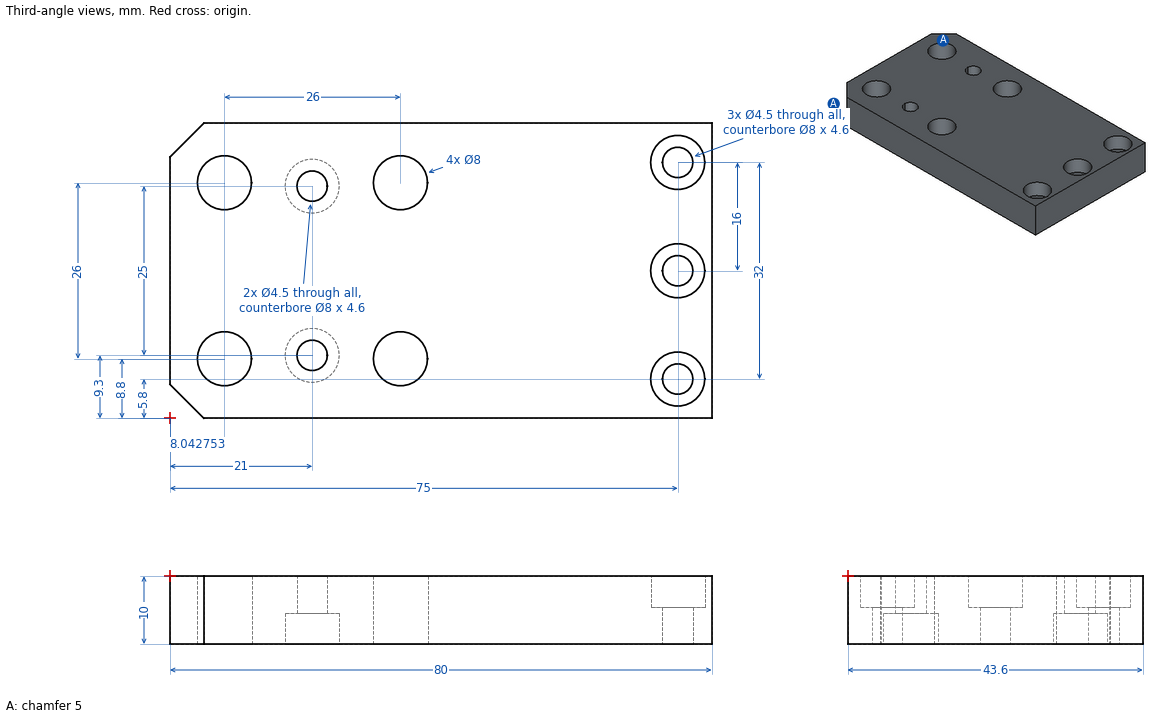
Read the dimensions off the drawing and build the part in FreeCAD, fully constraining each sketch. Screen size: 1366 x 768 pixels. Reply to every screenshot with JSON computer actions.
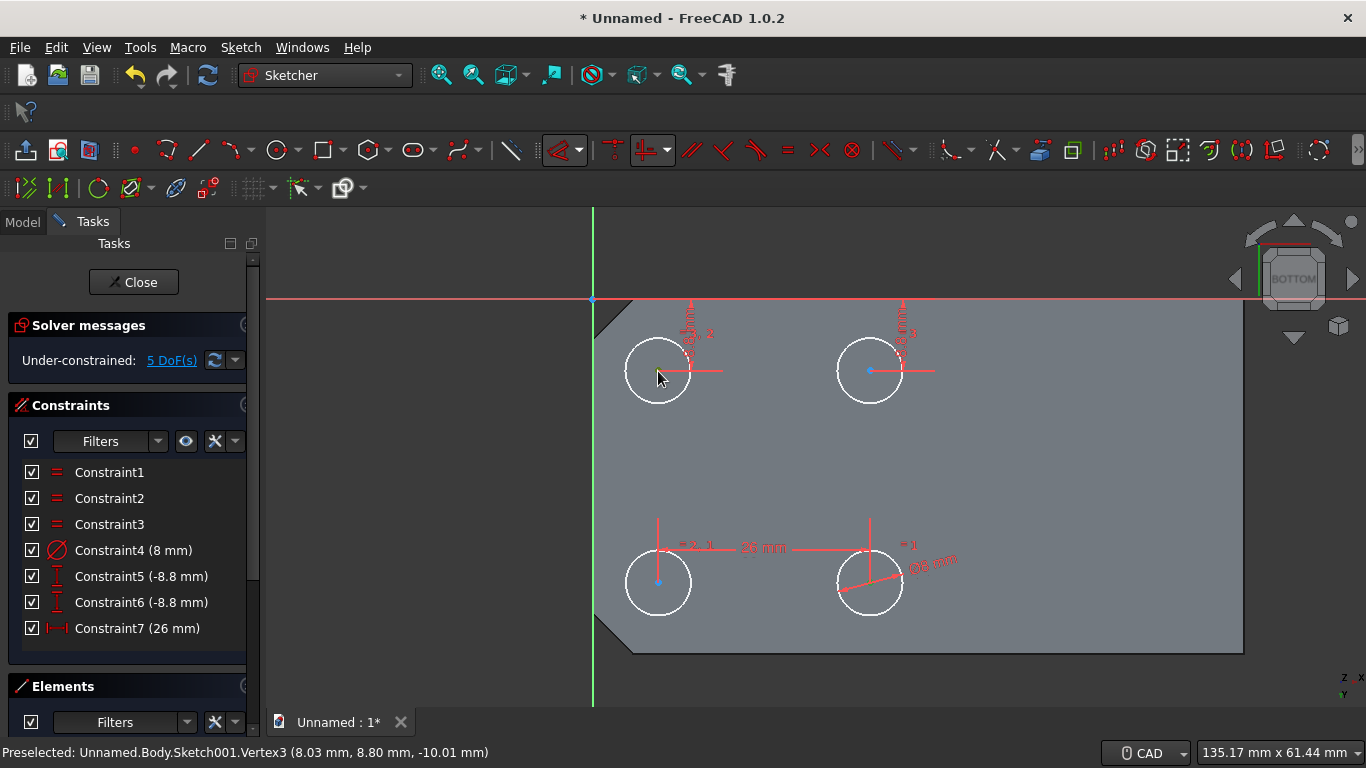
{"action": "left_click", "coordinate": [582, 150]}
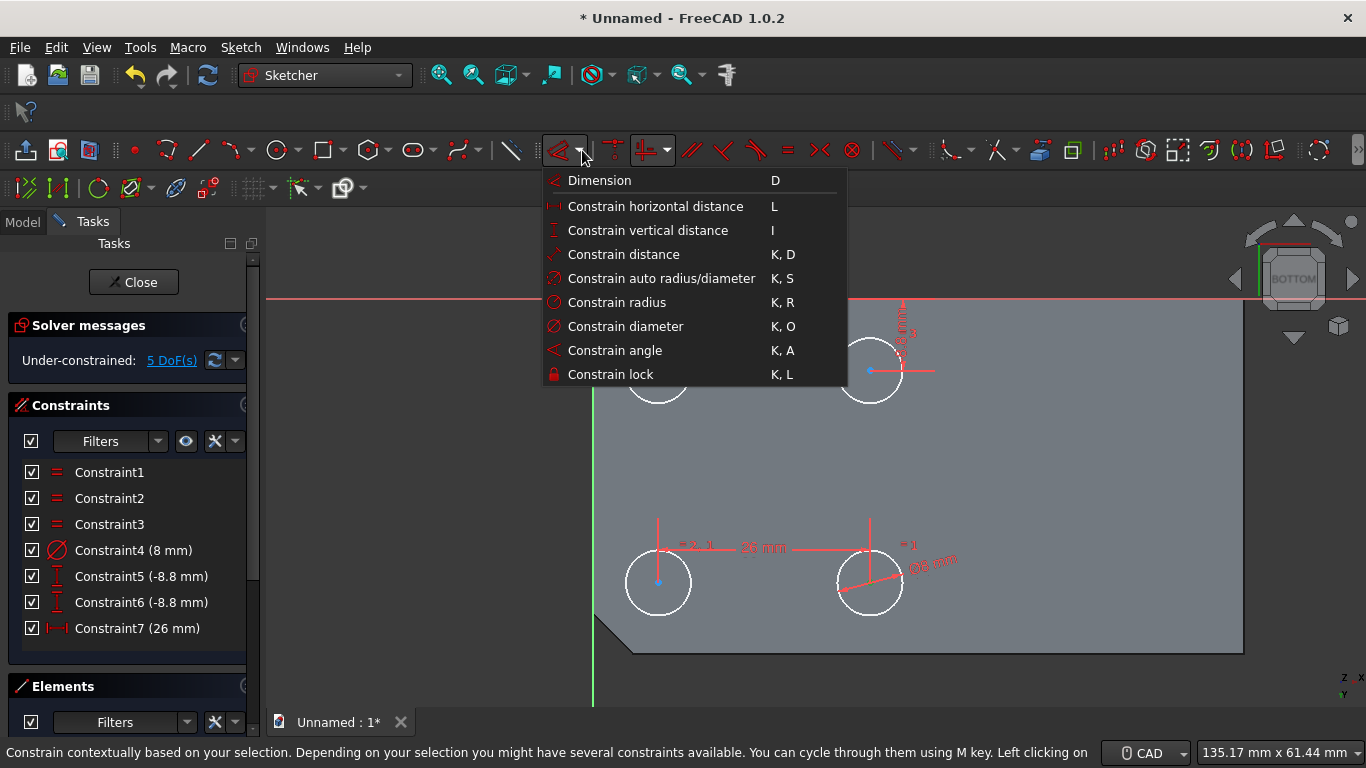
{"action": "left_click", "coordinate": [695, 206]}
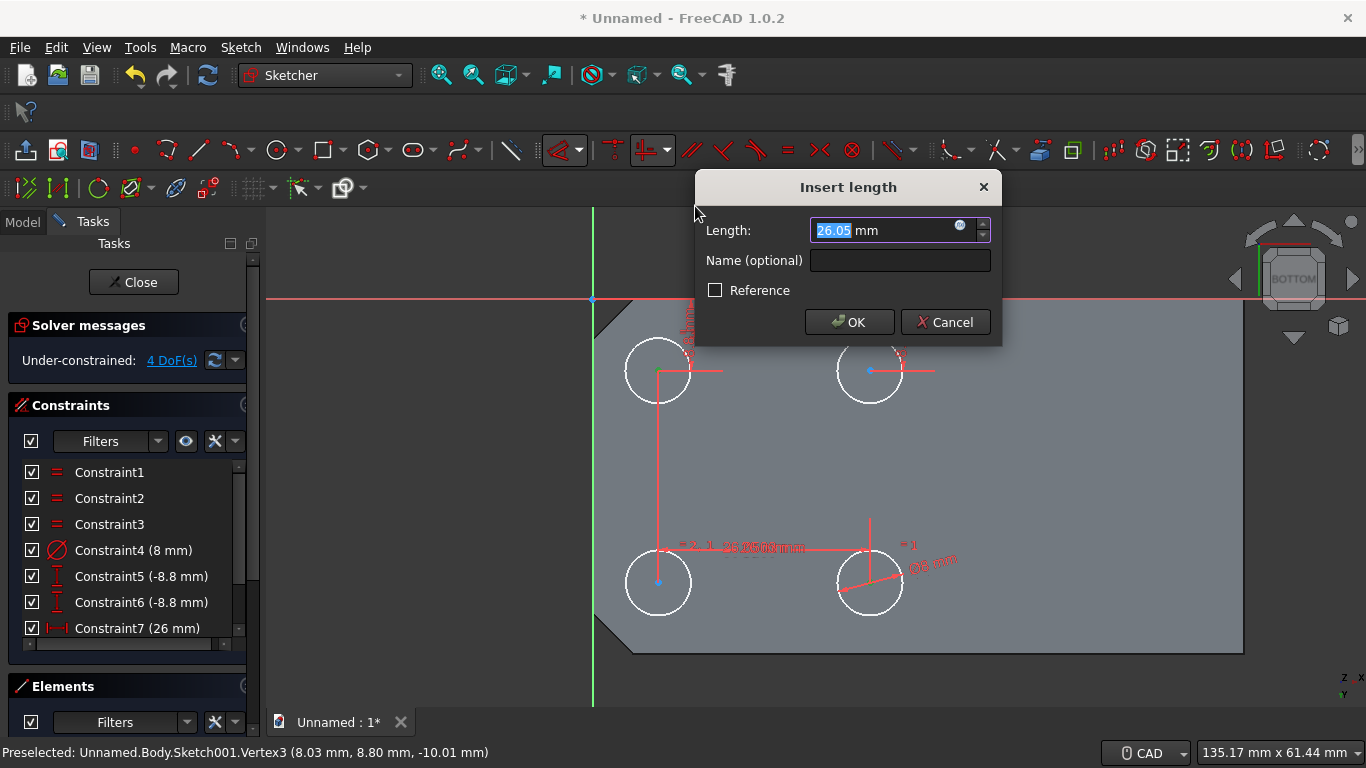
{"action": "type", "text": "26"}
{"action": "key", "text": "Return"}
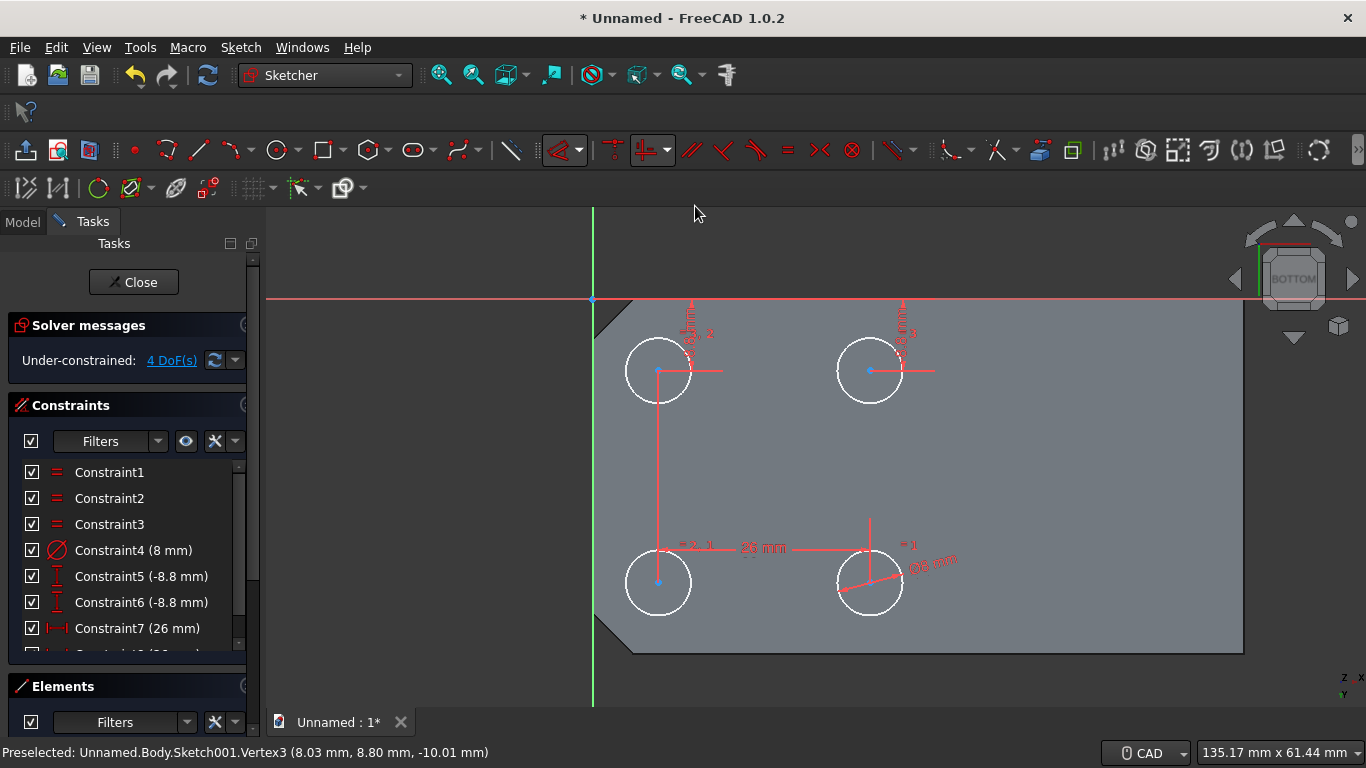
{"action": "left_click", "coordinate": [658, 583]}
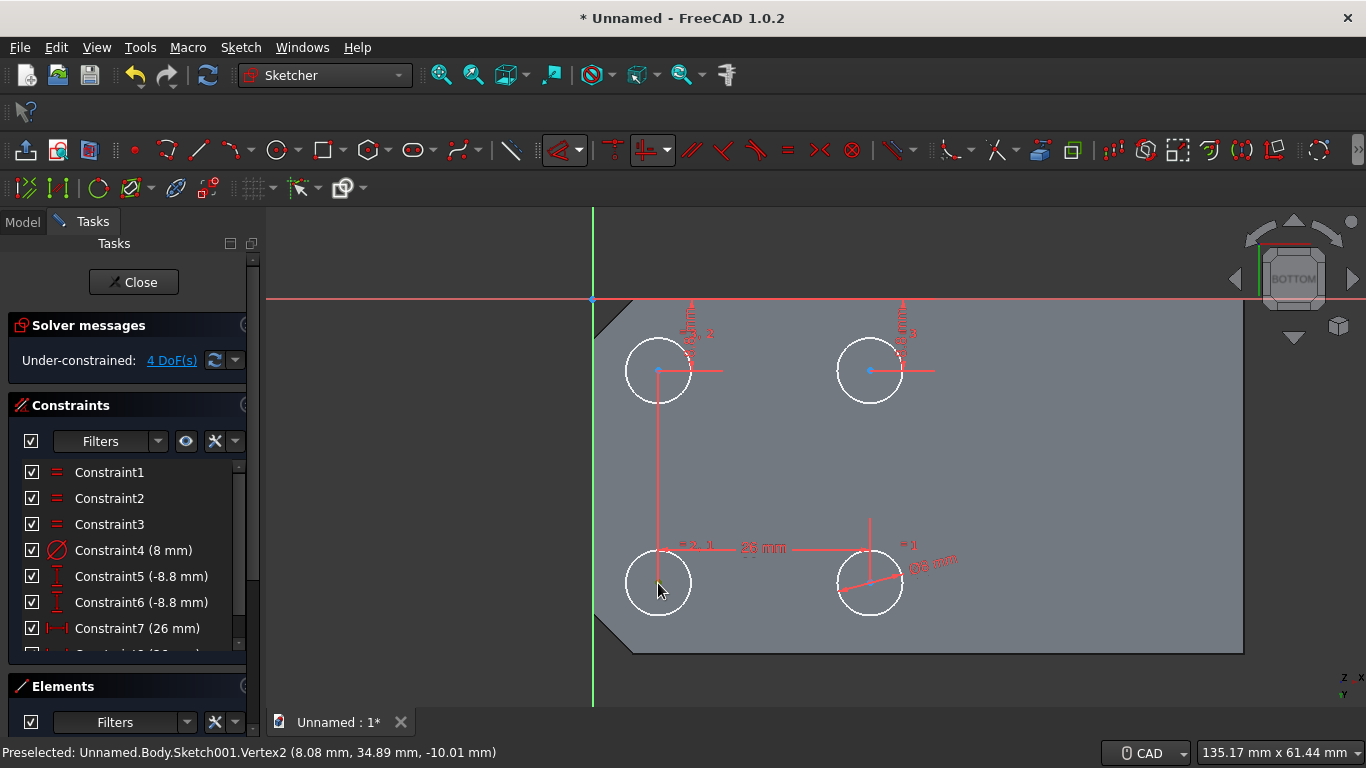
{"action": "left_click", "coordinate": [658, 371]}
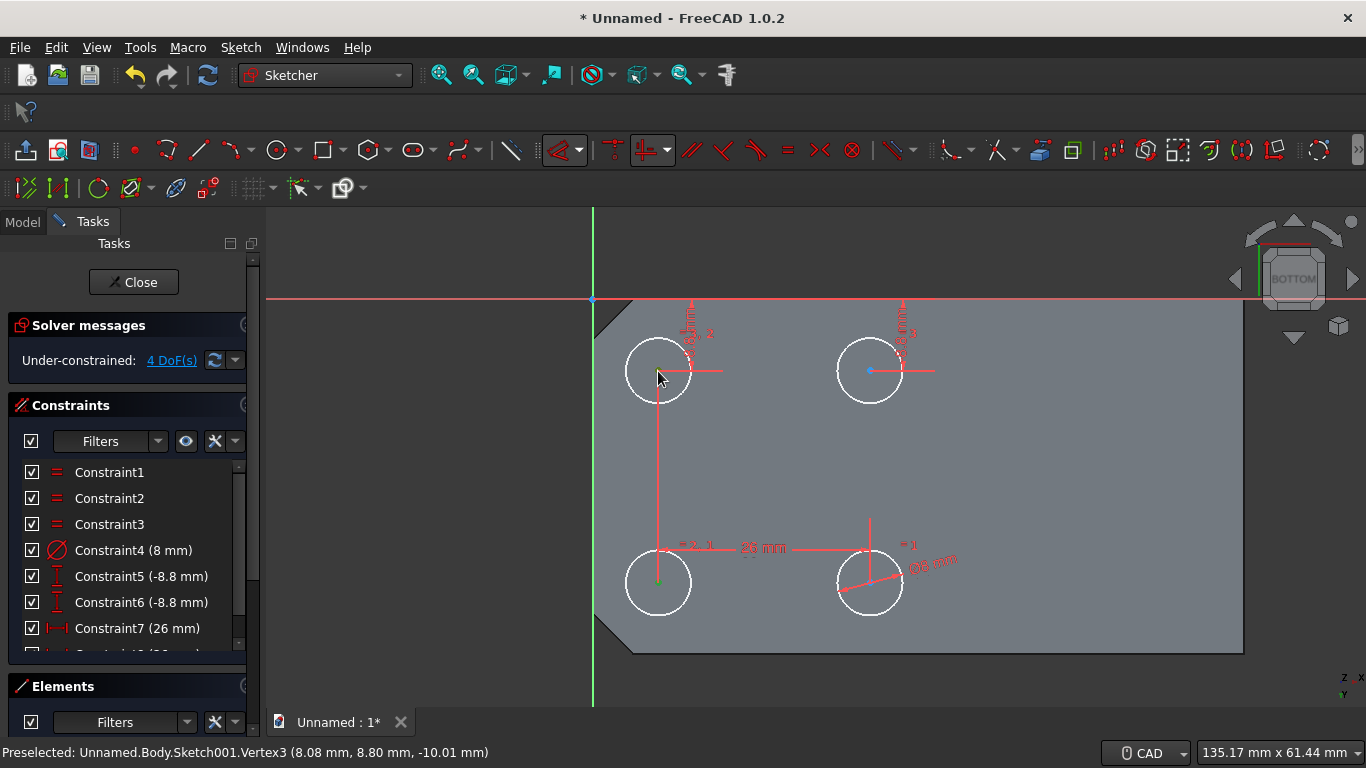
{"action": "key", "text": "i"}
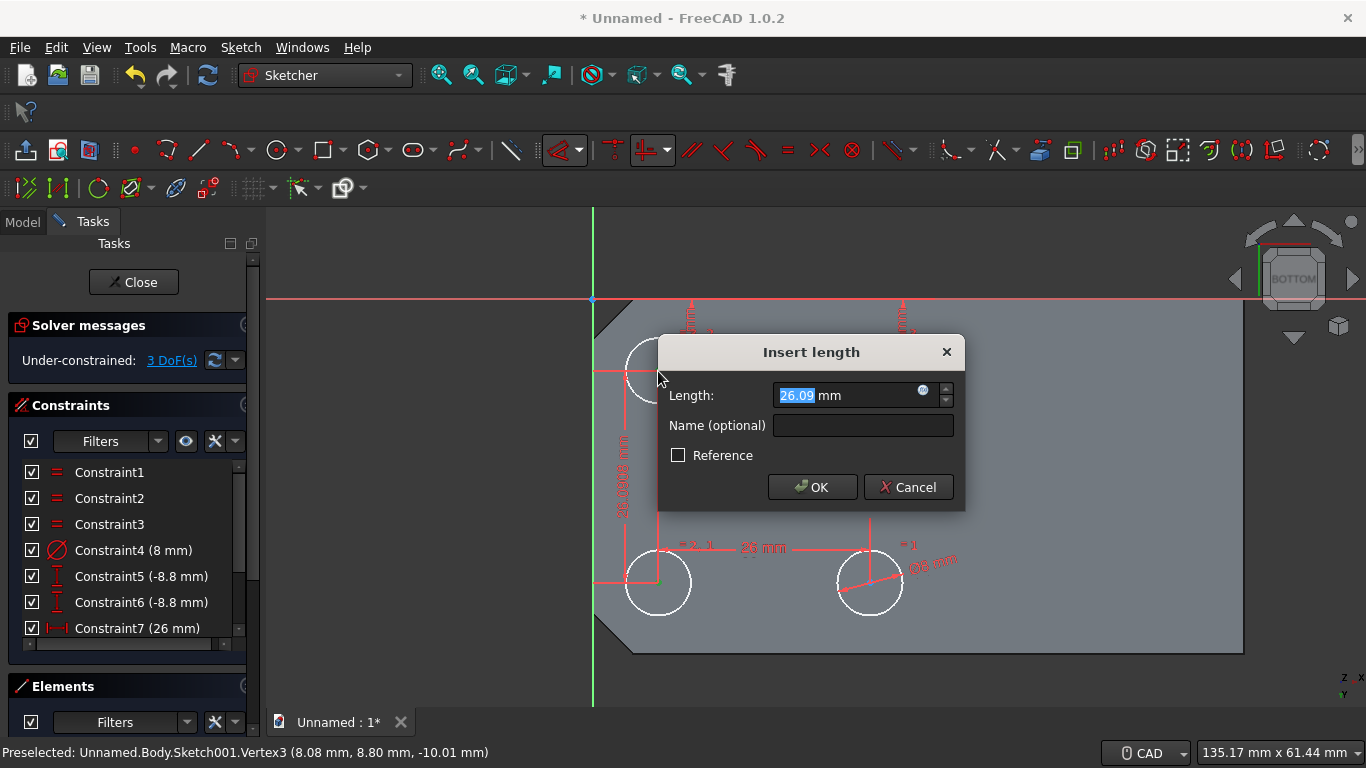
{"action": "type", "text": "26"}
{"action": "key", "text": "Return"}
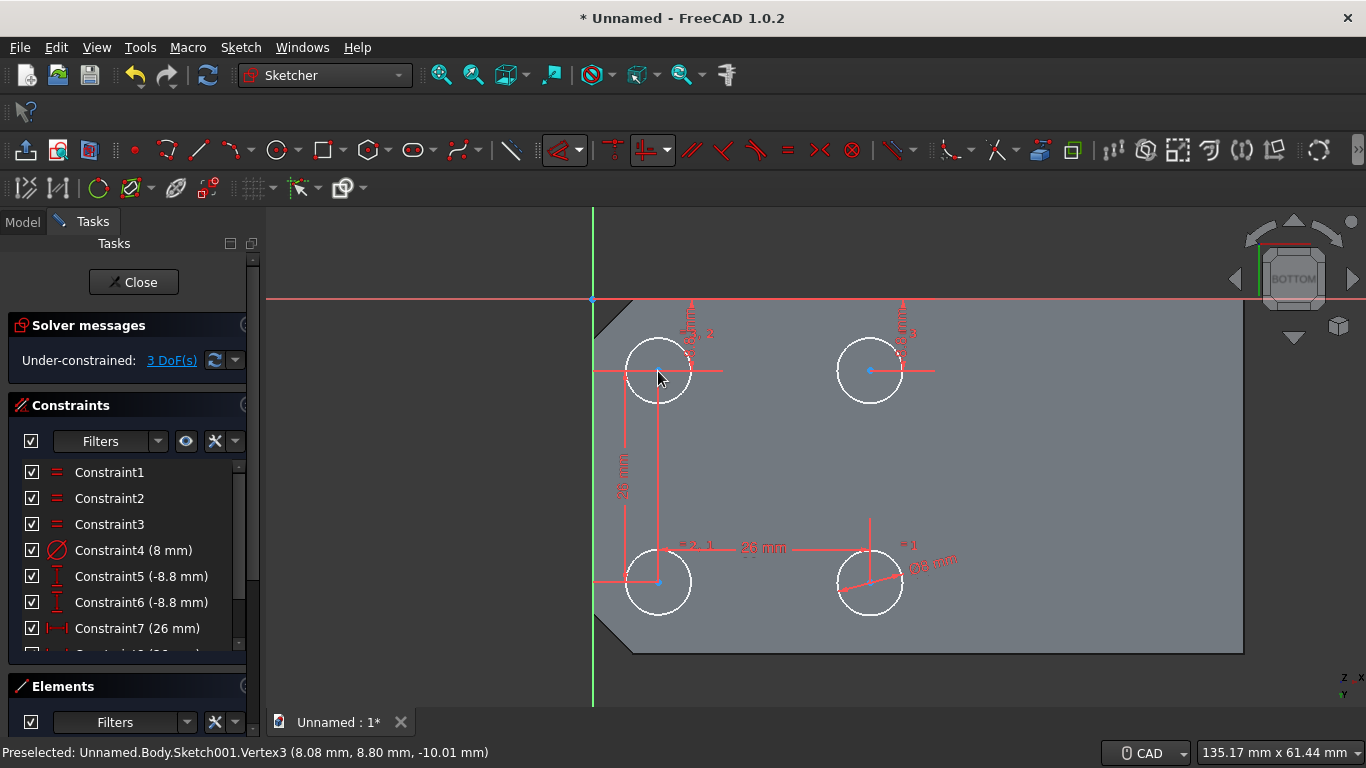
{"action": "left_click", "coordinate": [870, 583]}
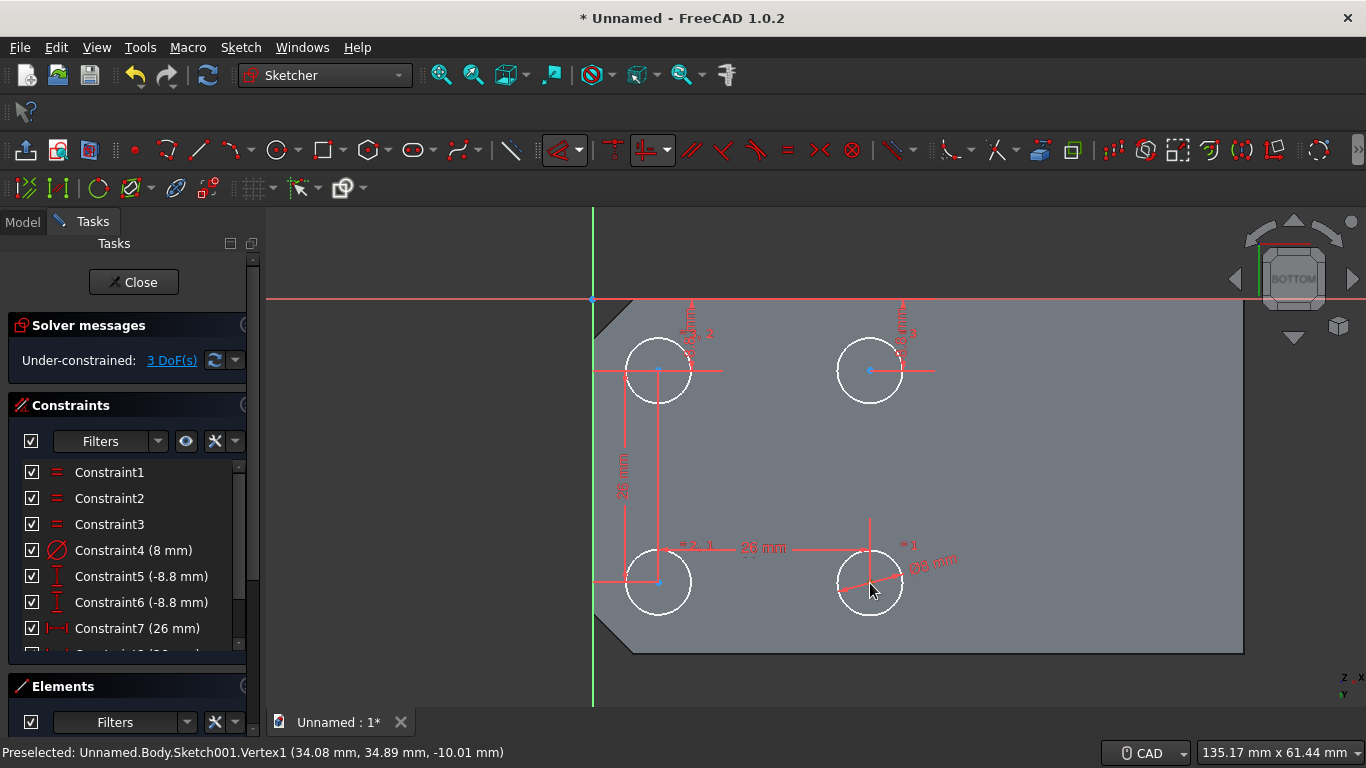
{"action": "left_click", "coordinate": [658, 371]}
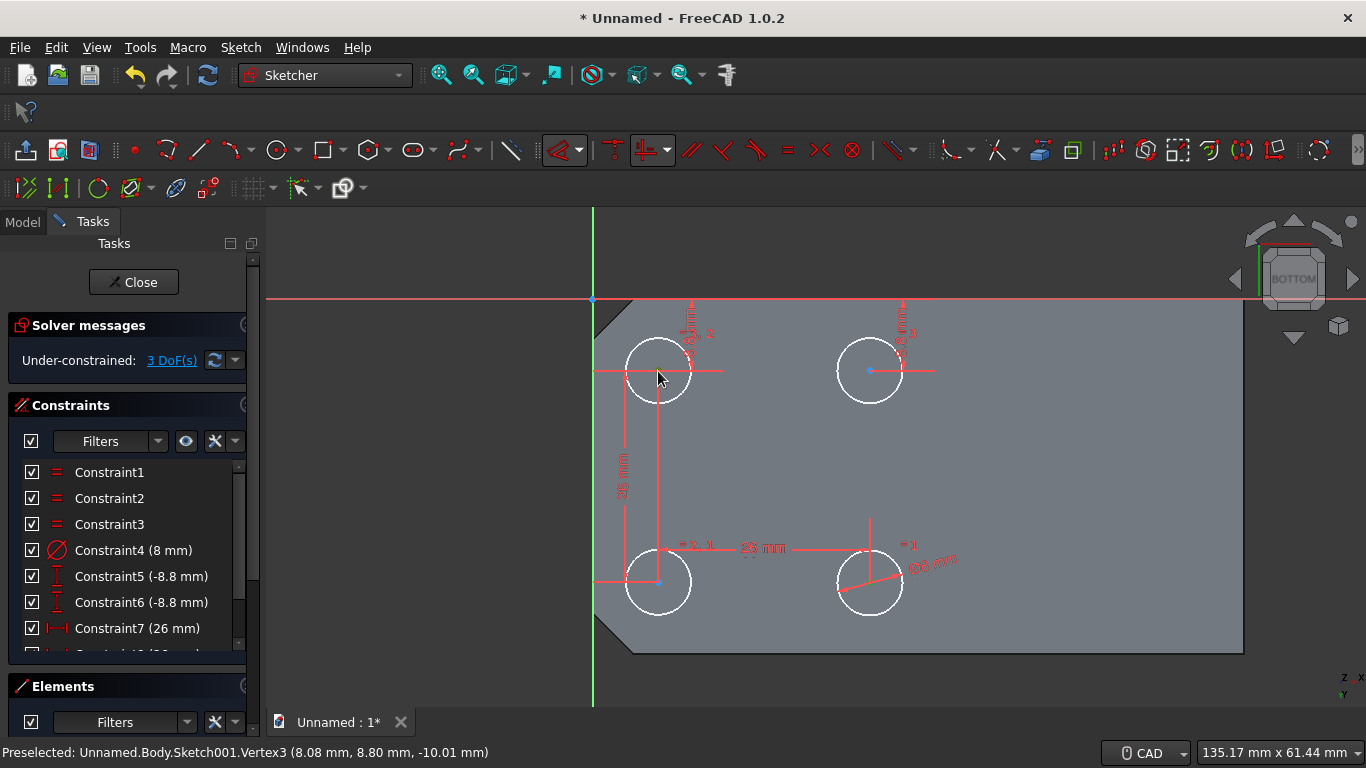
{"action": "key", "text": "i"}